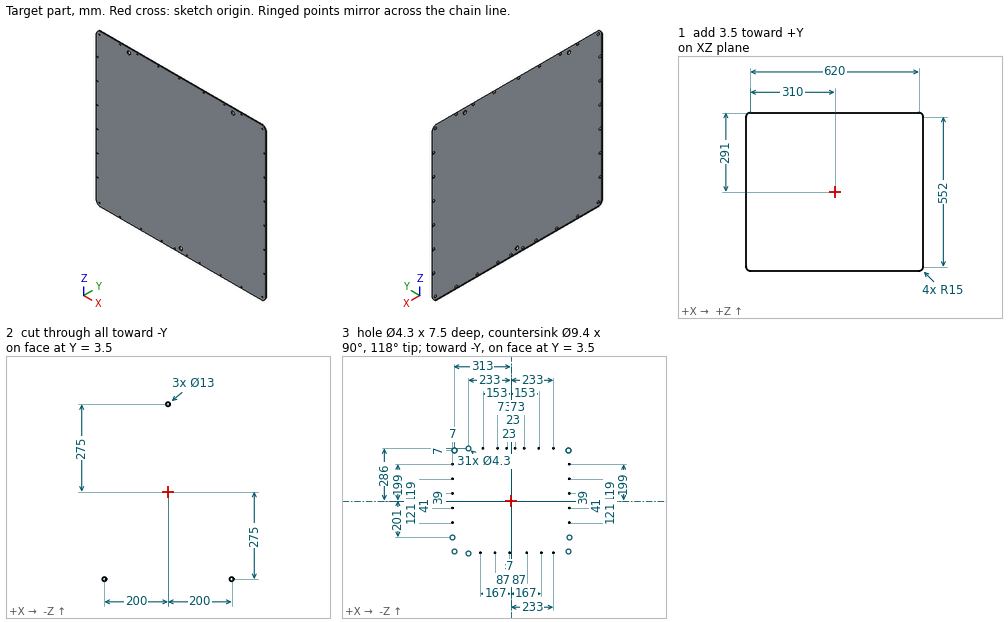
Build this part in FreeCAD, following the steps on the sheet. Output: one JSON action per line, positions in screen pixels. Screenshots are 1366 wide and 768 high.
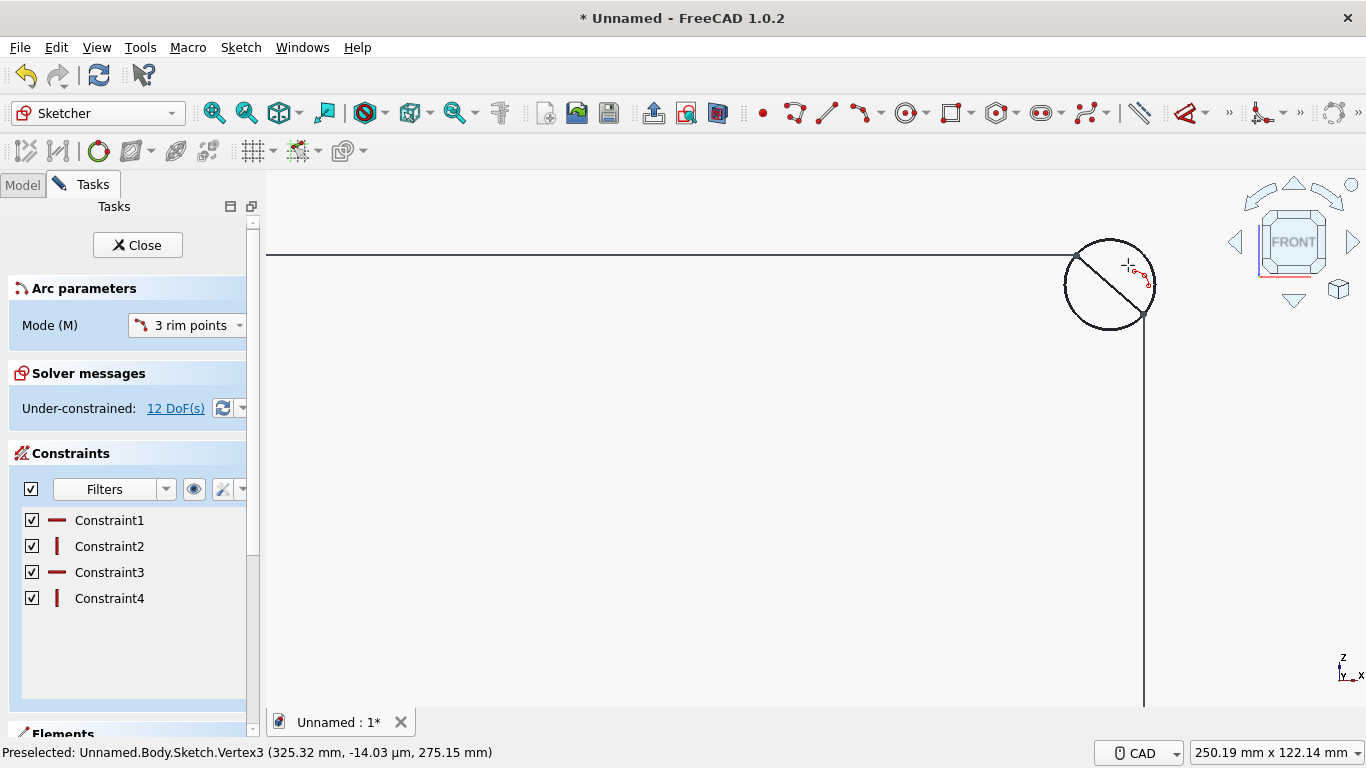
{"action": "left_click", "coordinate": [1123, 264]}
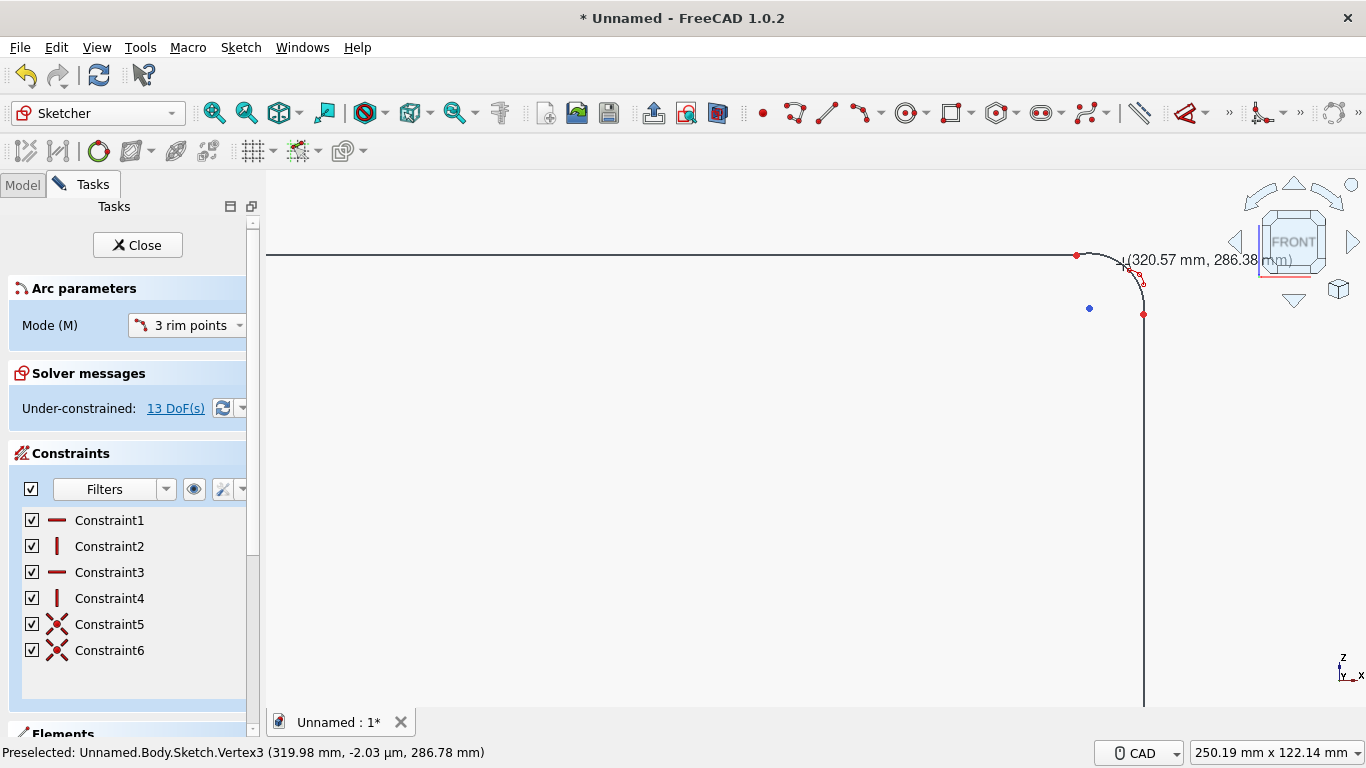
{"action": "scroll", "coordinate": [909, 269], "scroll_direction": "down", "scroll_amount": 10}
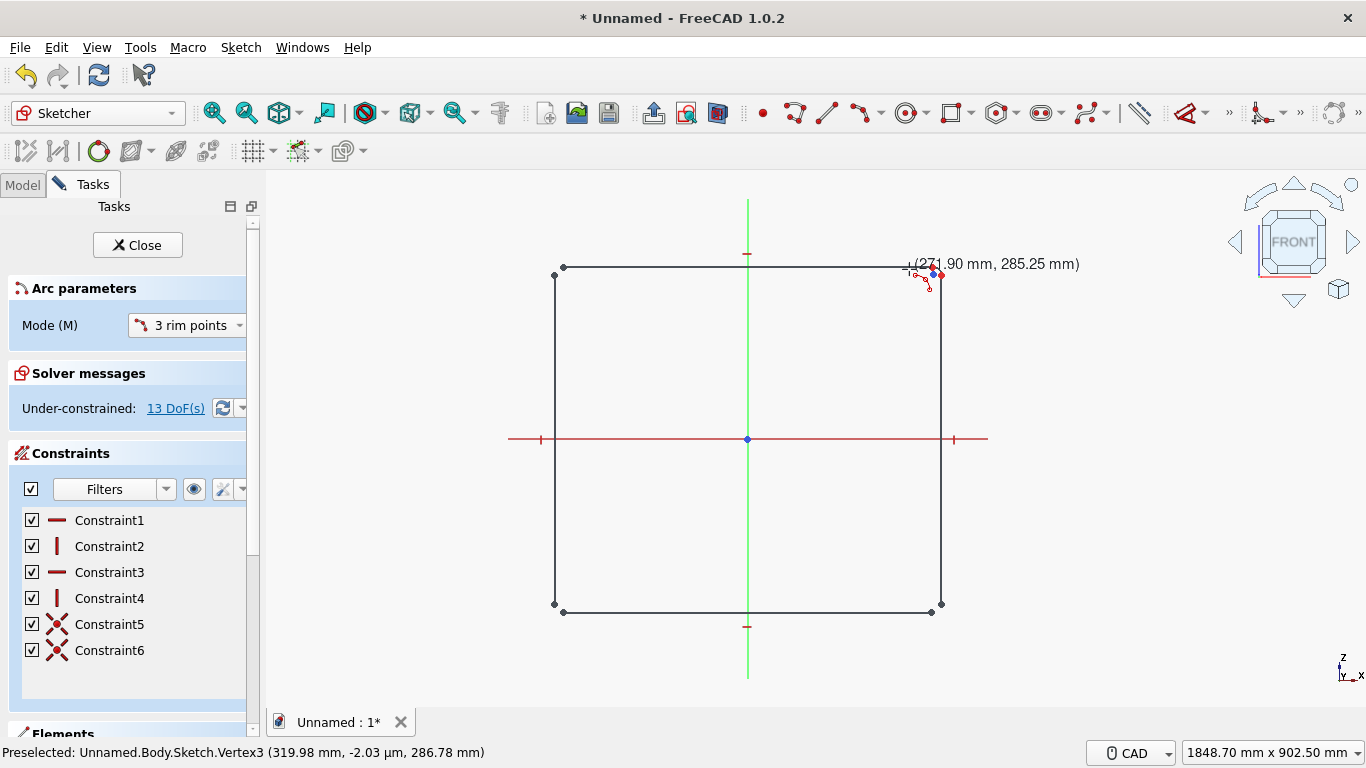
{"action": "scroll", "coordinate": [941, 603], "scroll_direction": "up", "scroll_amount": 2}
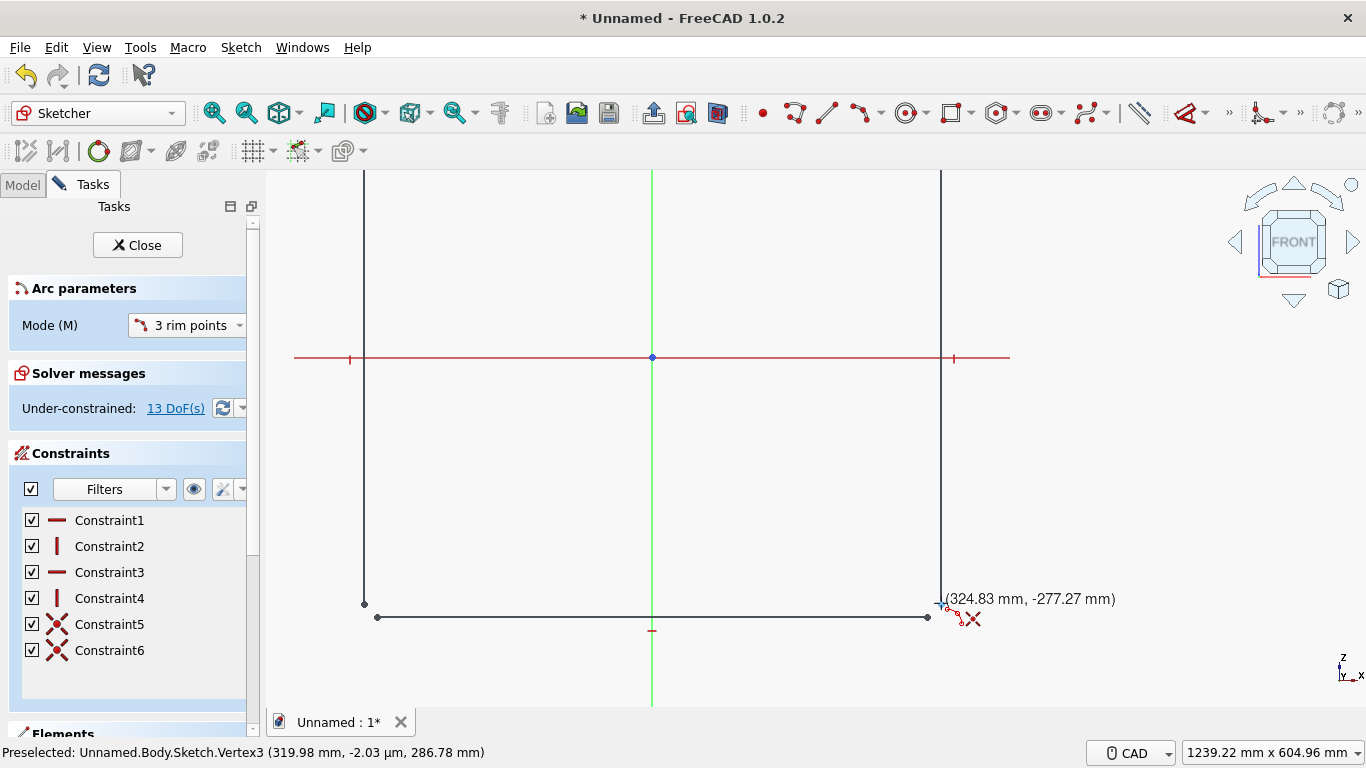
{"action": "left_click", "coordinate": [941, 604]}
{"action": "left_click", "coordinate": [927, 617]}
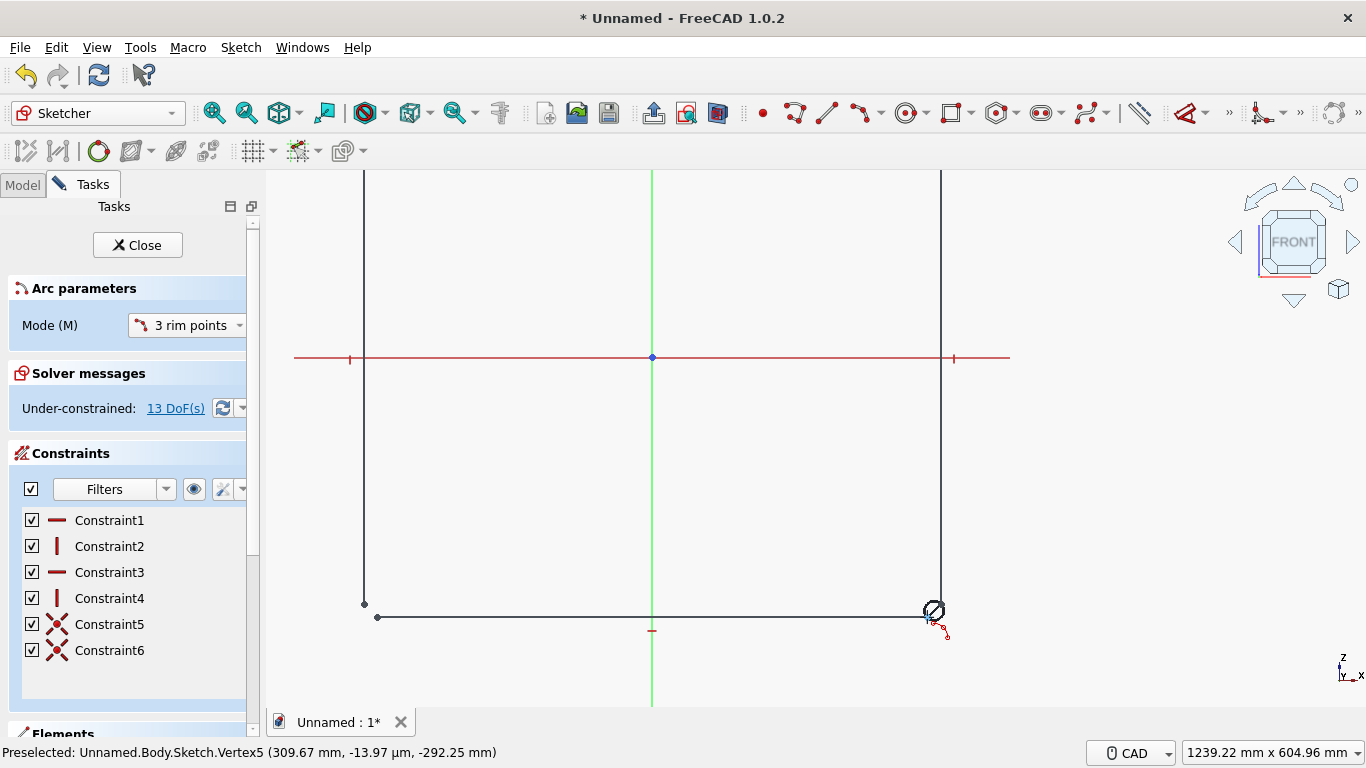
{"action": "scroll", "coordinate": [937, 612], "scroll_direction": "up", "scroll_amount": 8}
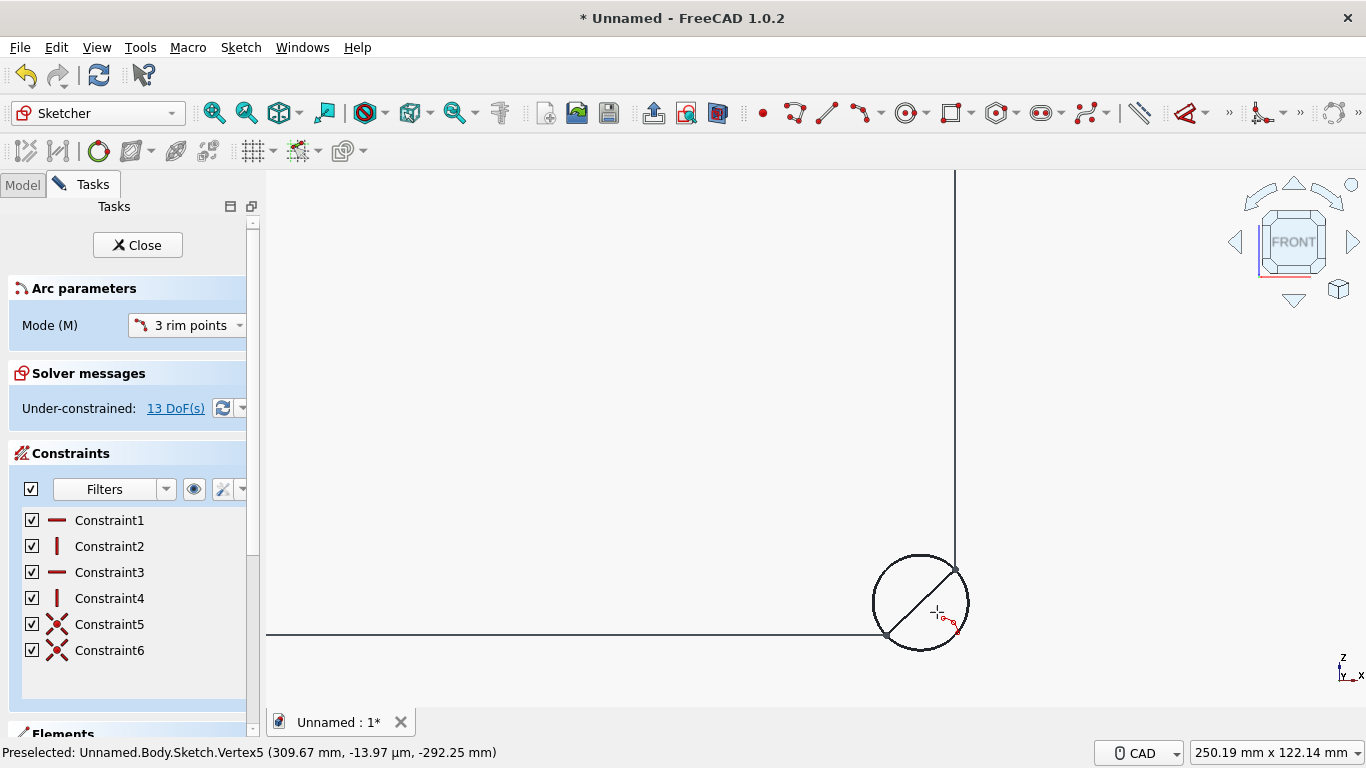
{"action": "left_click", "coordinate": [934, 611]}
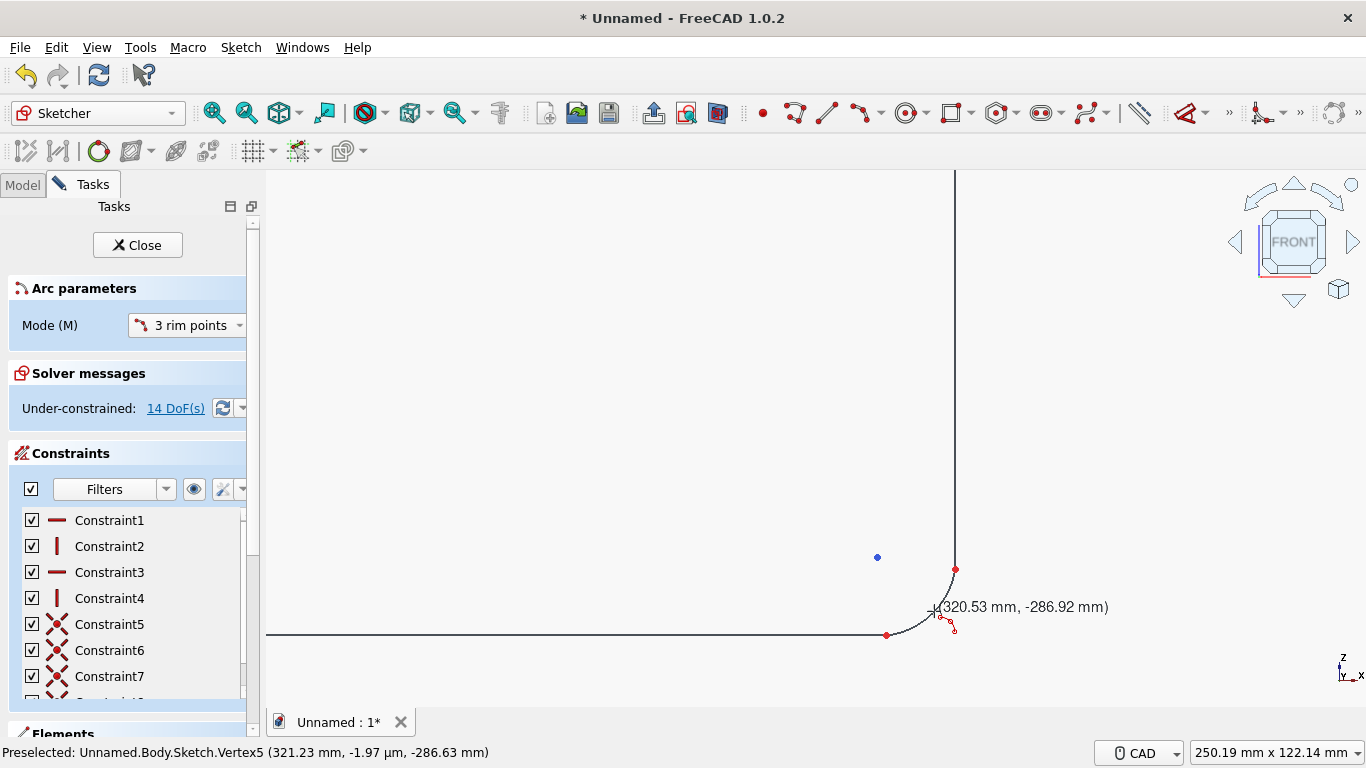
{"action": "scroll", "coordinate": [939, 609], "scroll_direction": "down", "scroll_amount": 10}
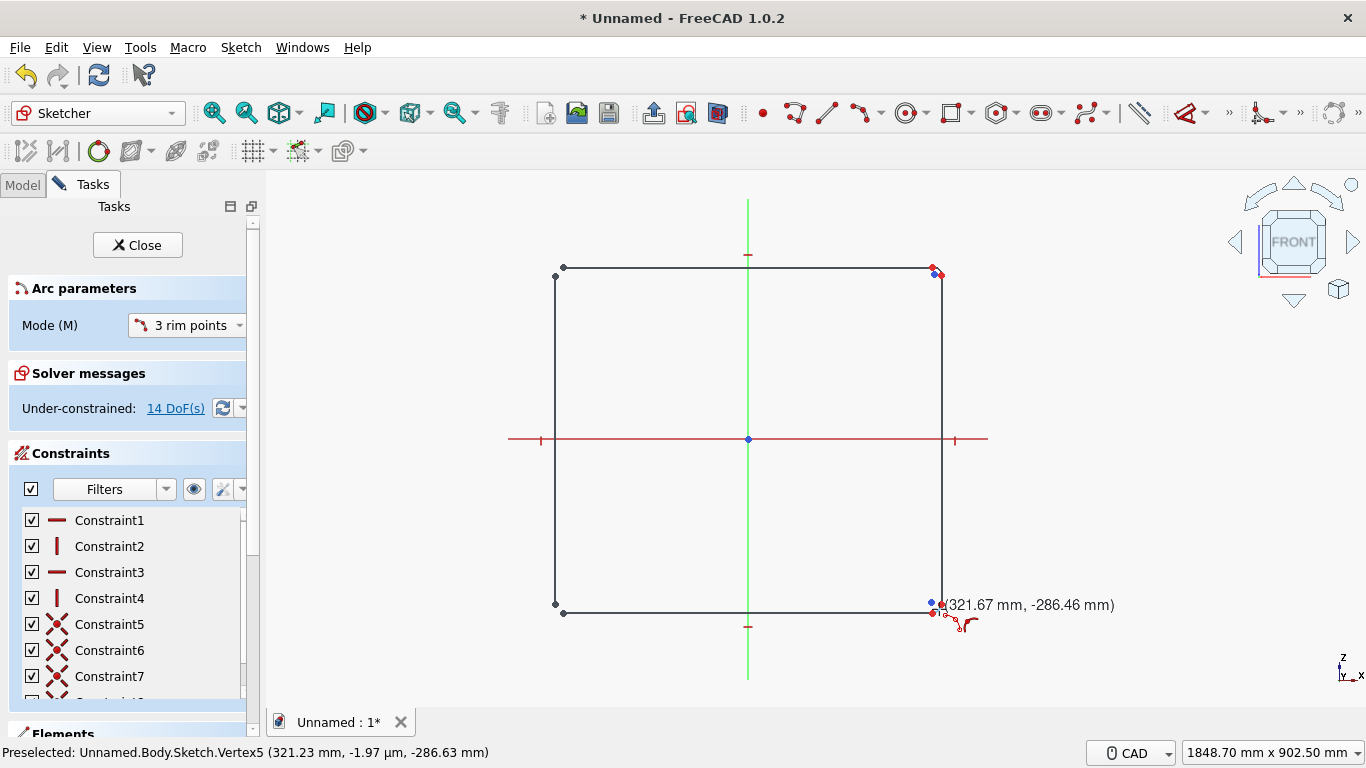
{"action": "scroll", "coordinate": [564, 613], "scroll_direction": "up", "scroll_amount": 2}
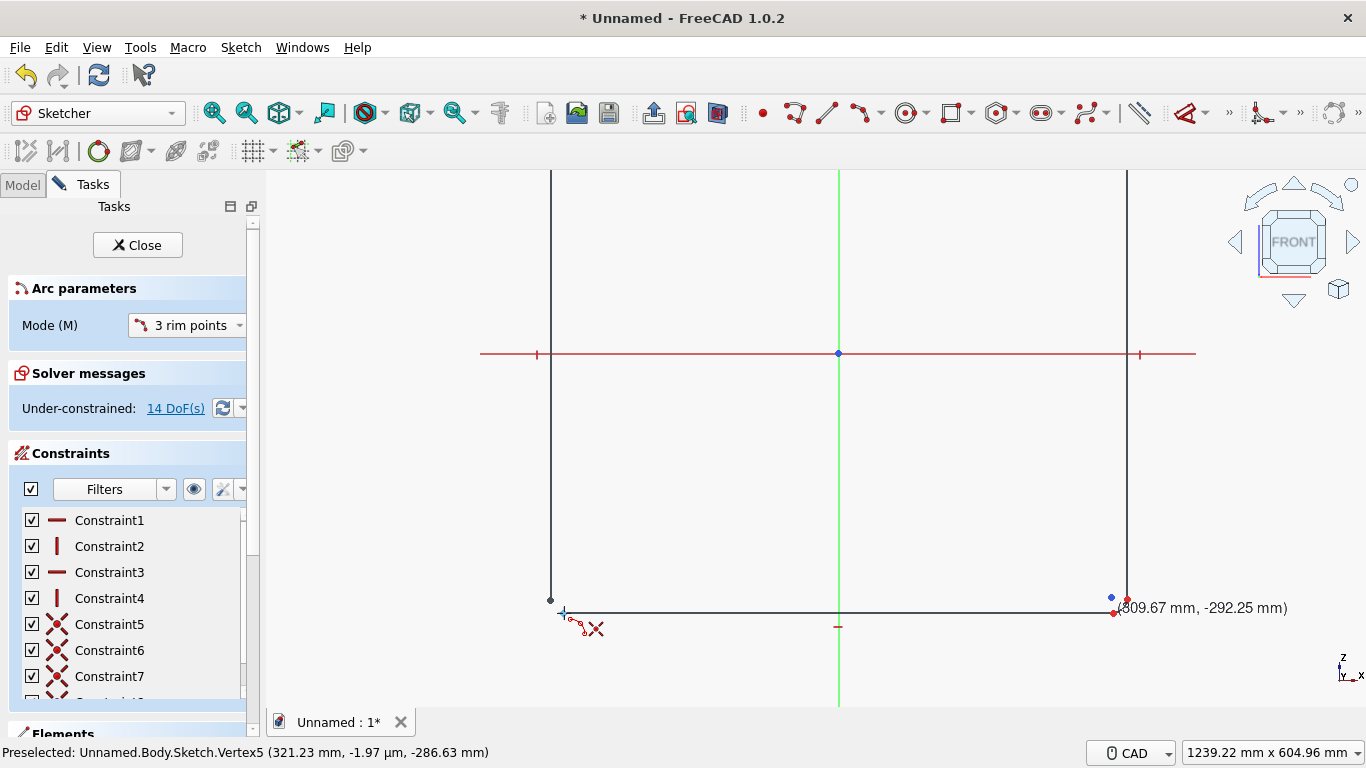
{"action": "left_click", "coordinate": [563, 613]}
{"action": "left_click", "coordinate": [551, 600]}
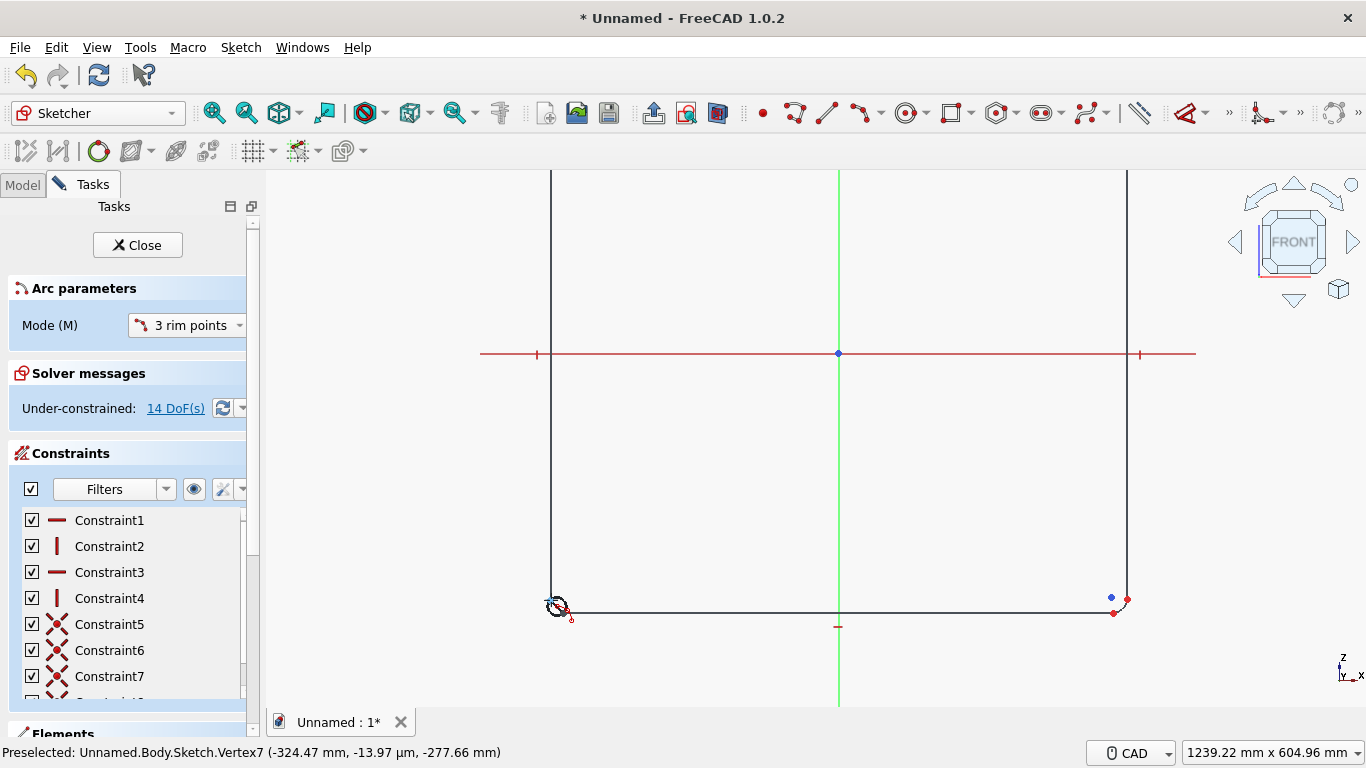
{"action": "scroll", "coordinate": [554, 608], "scroll_direction": "up", "scroll_amount": 8}